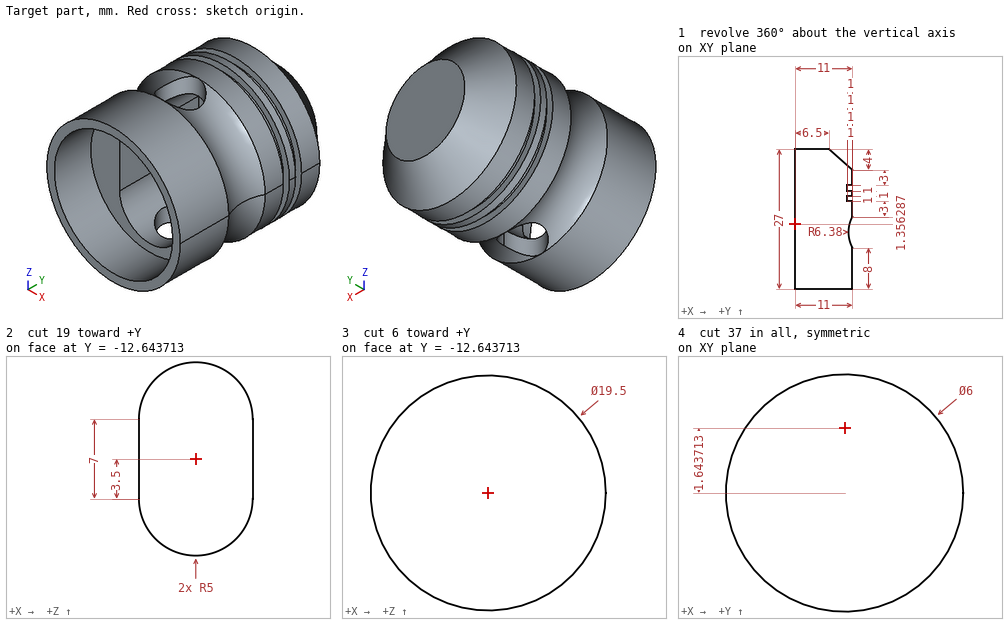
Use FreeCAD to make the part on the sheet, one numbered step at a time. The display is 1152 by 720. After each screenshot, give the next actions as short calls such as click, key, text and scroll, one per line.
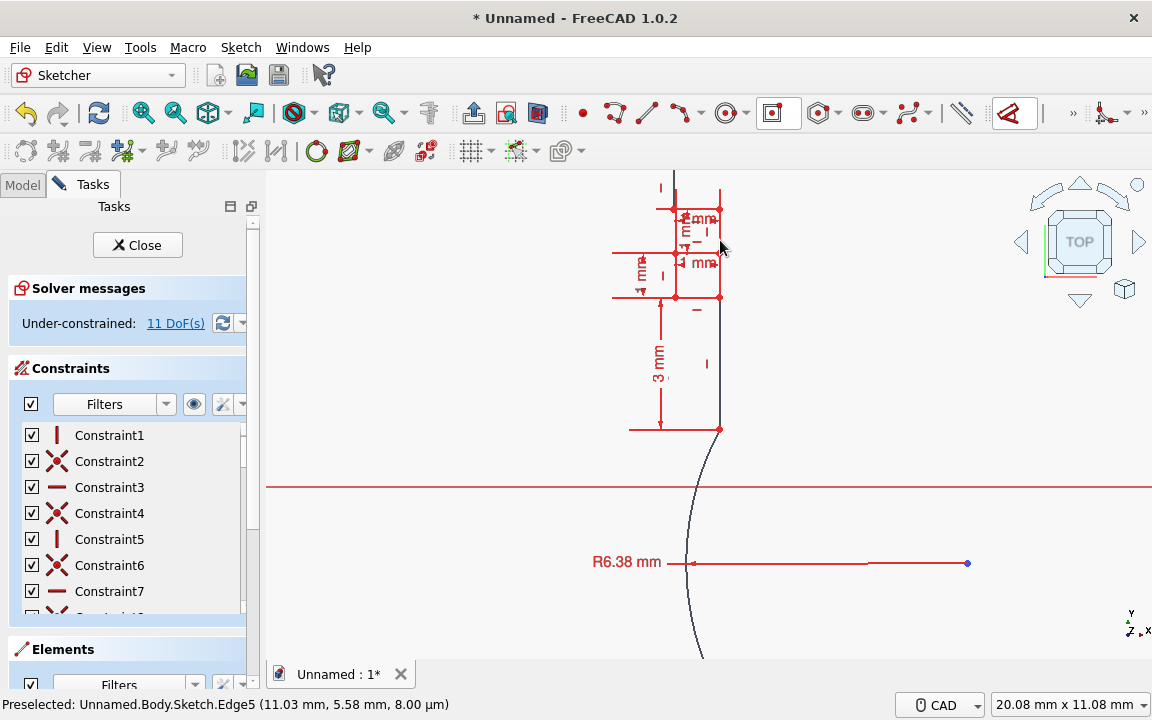
click(706, 209)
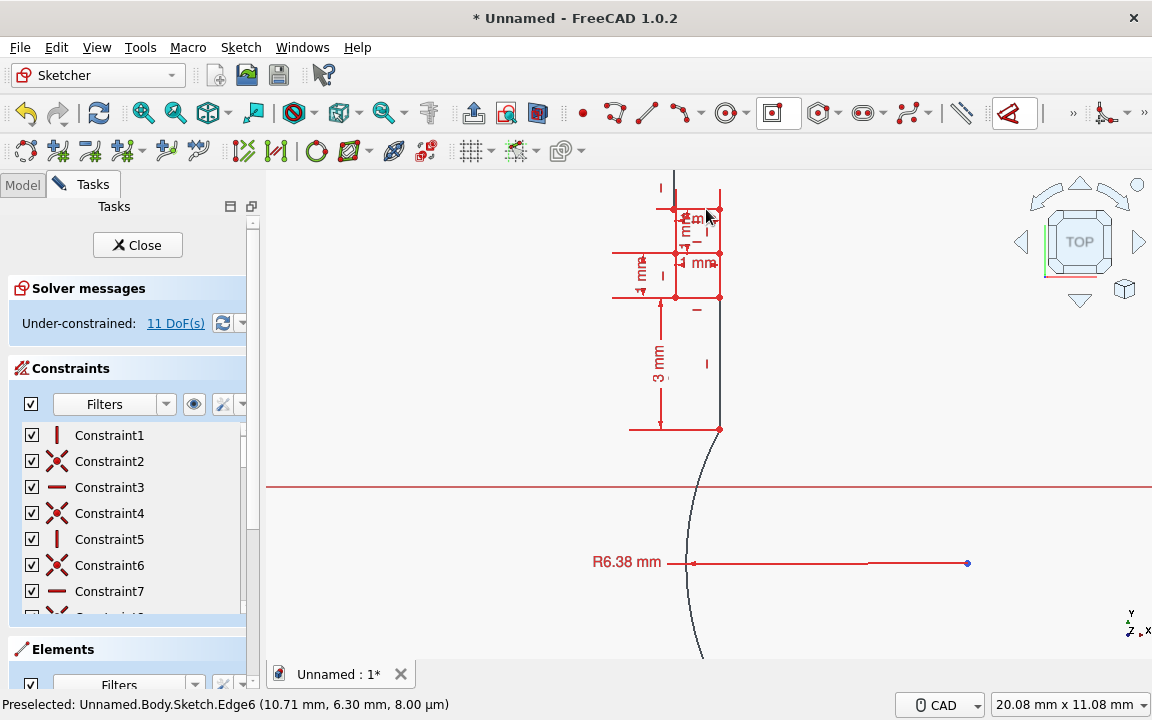
click(1032, 114)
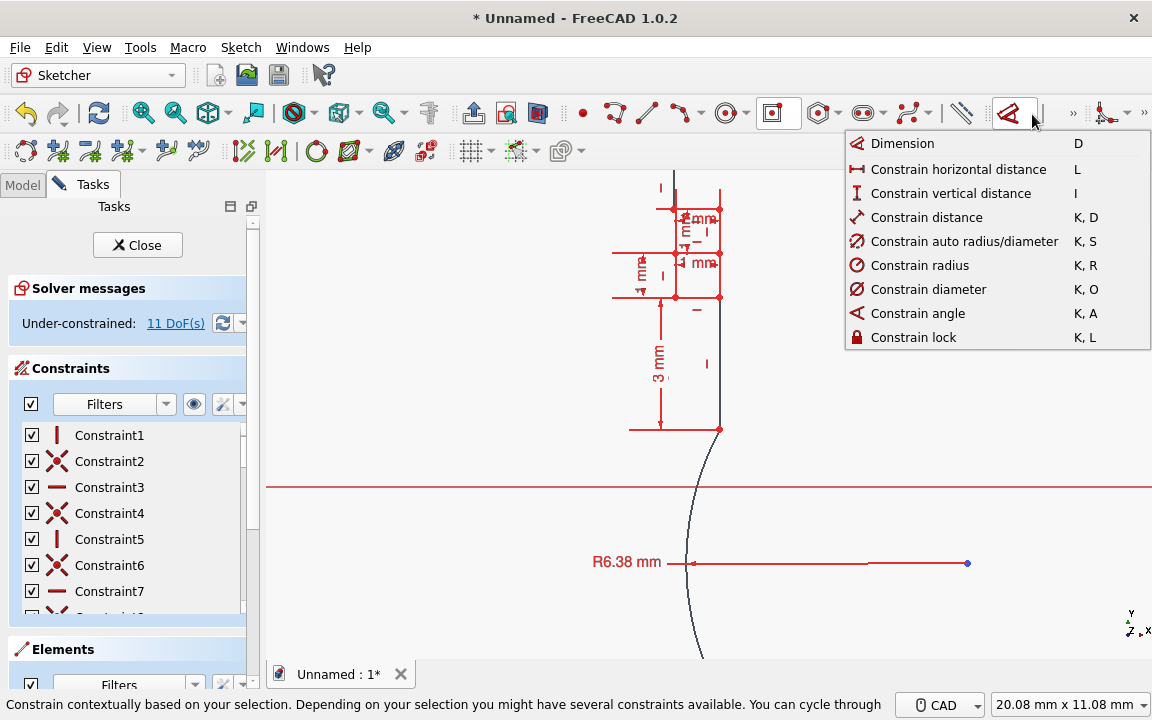
click(998, 169)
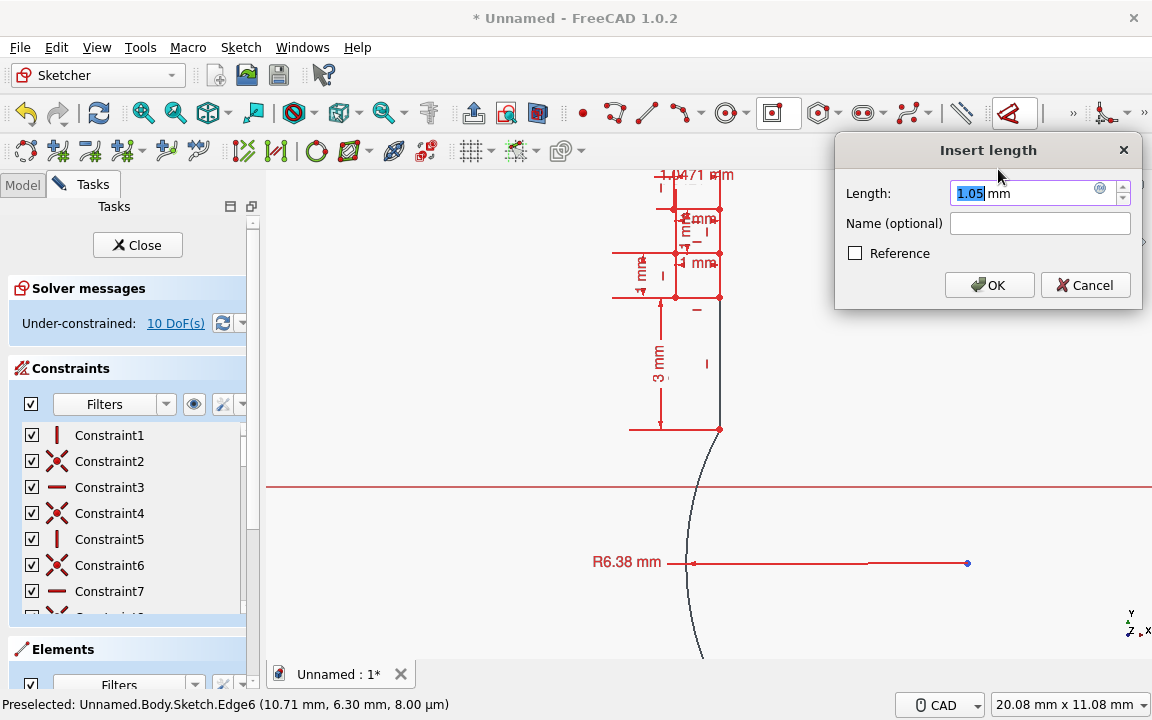
text(1)
key(Return)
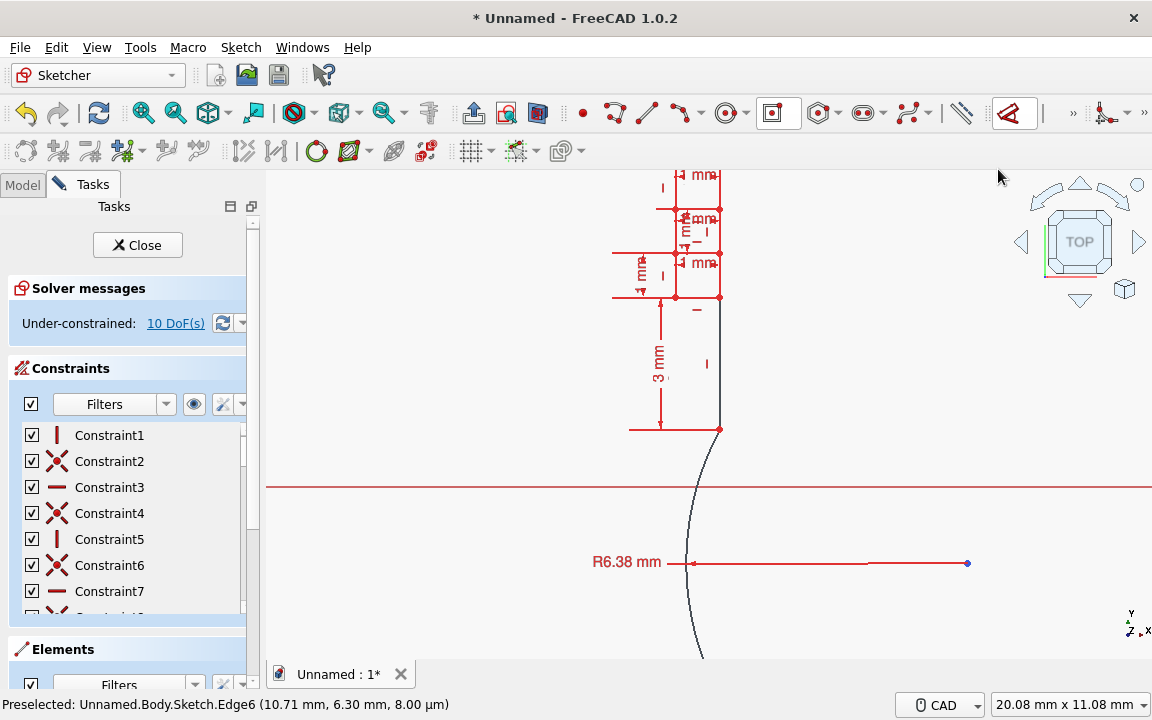
scroll(694, 403, down, 7)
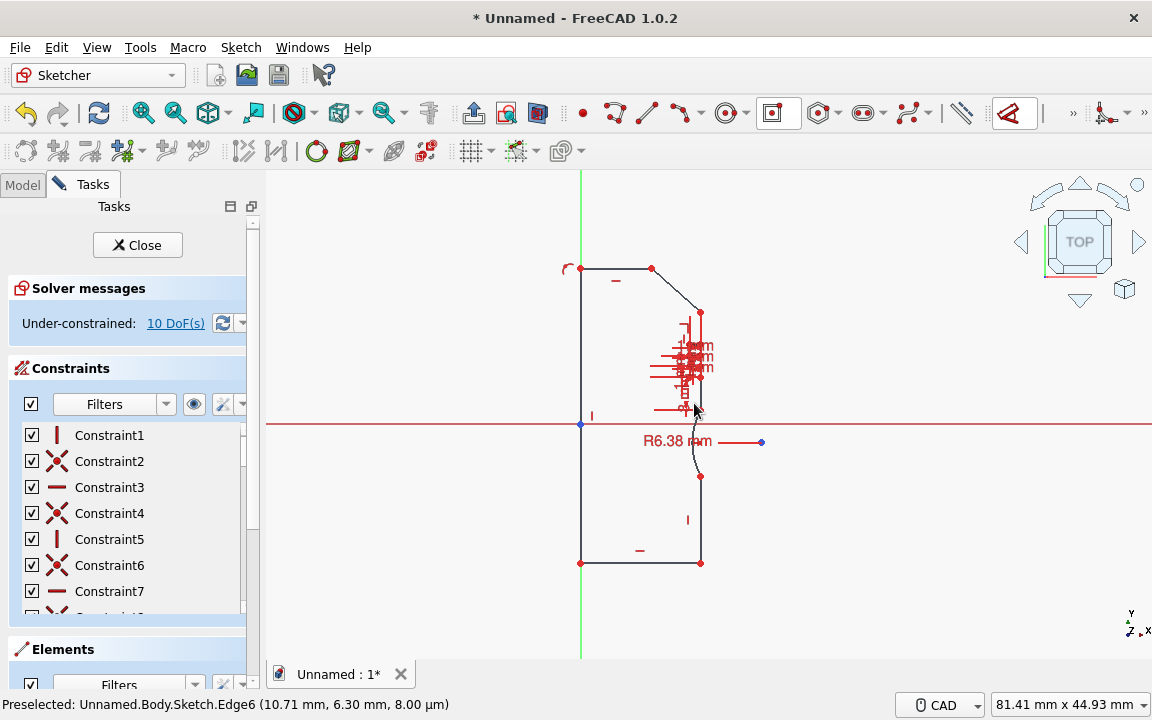
scroll(690, 352, up, 8)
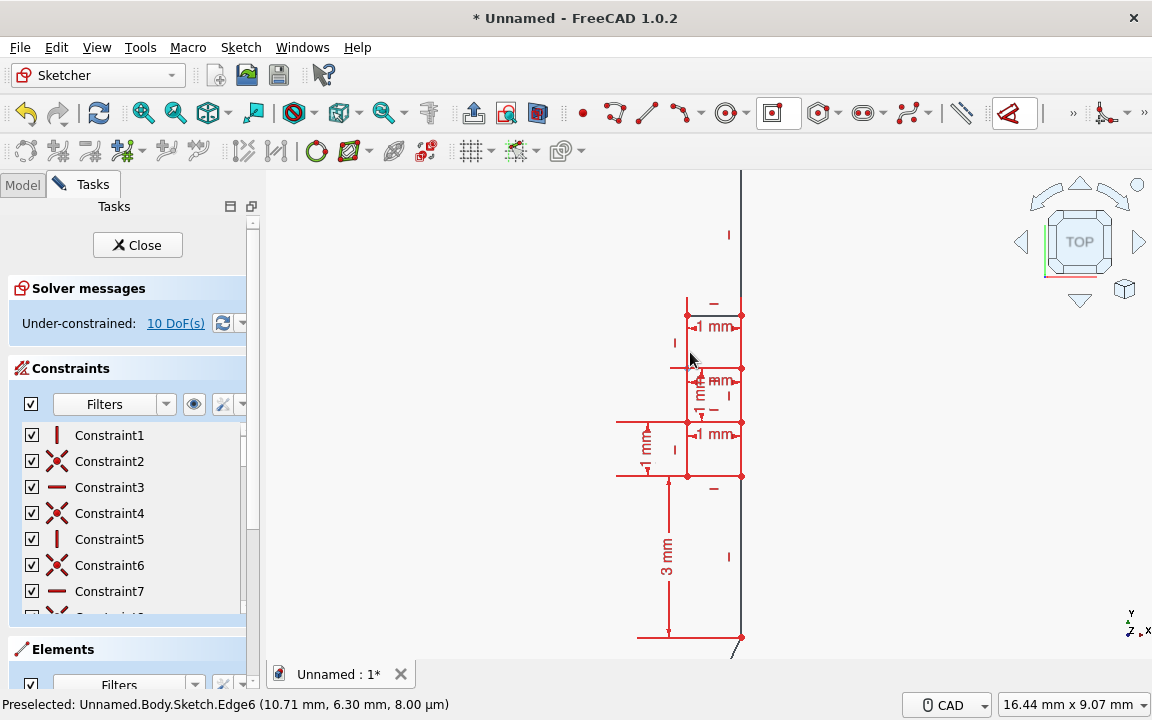
click(687, 353)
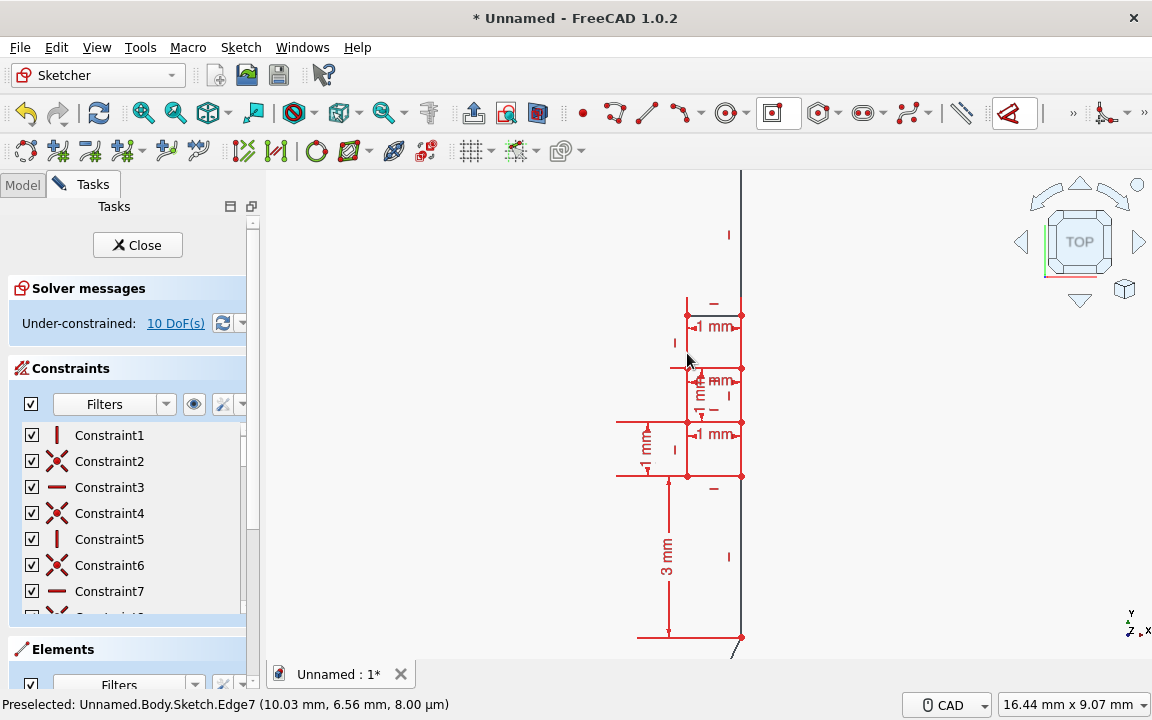
click(1032, 114)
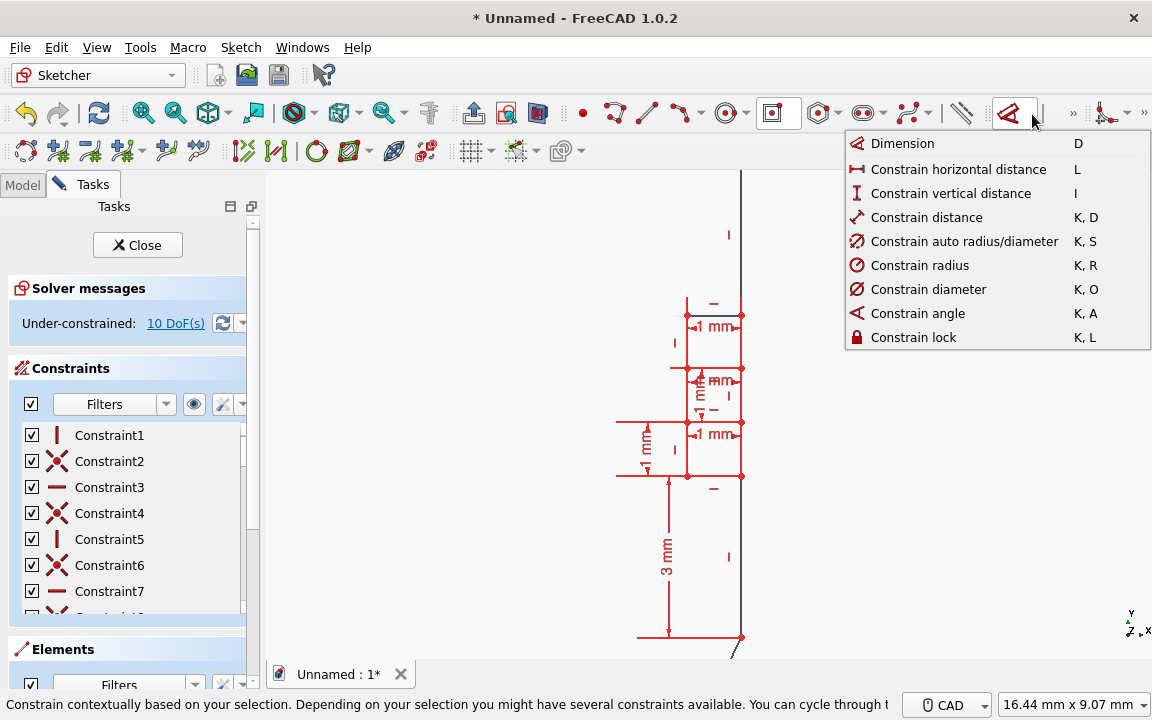
click(998, 193)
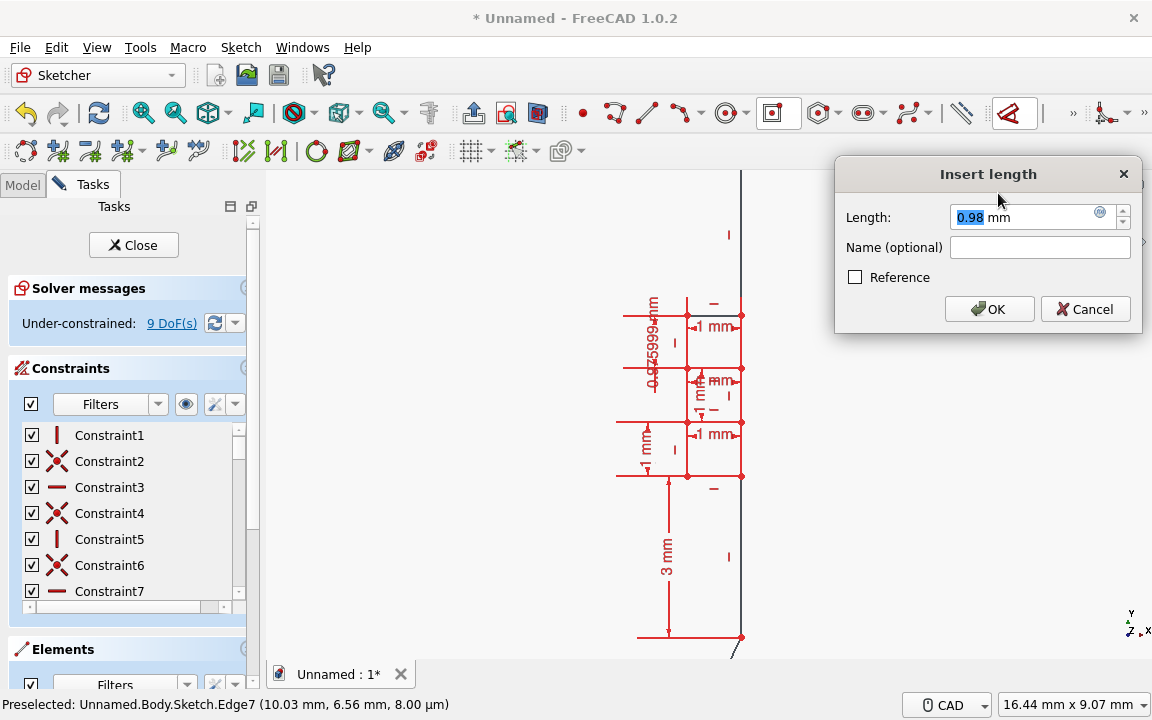
text(1)
key(Return)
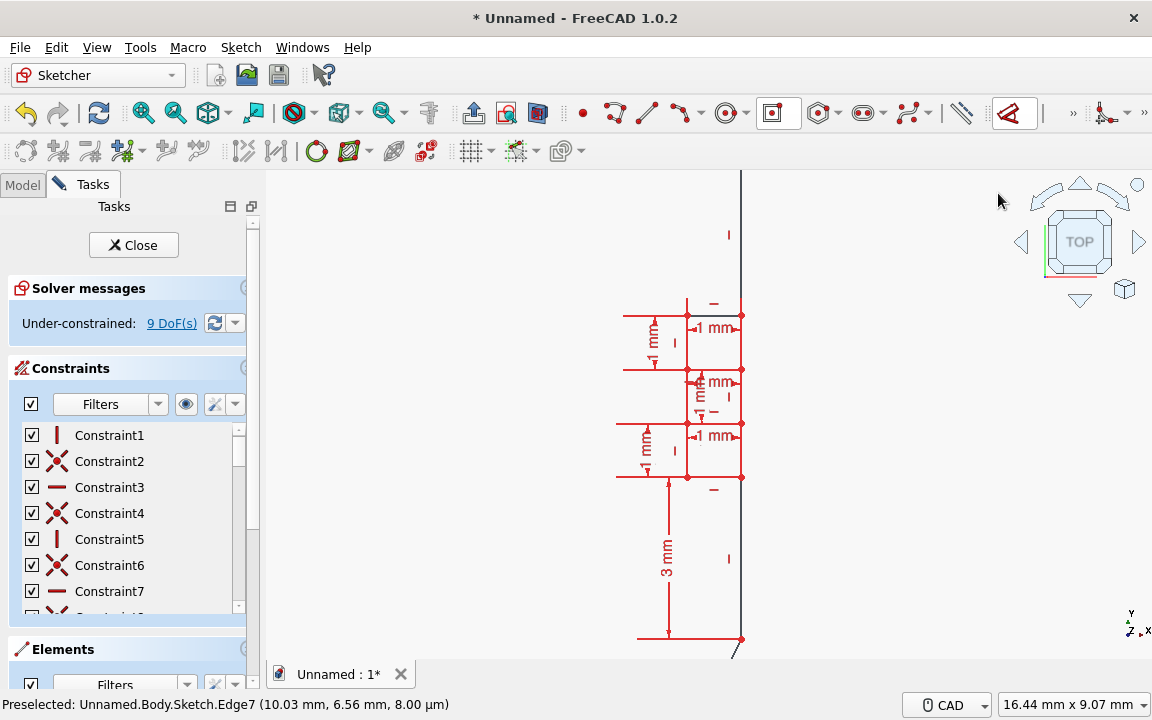
click(704, 316)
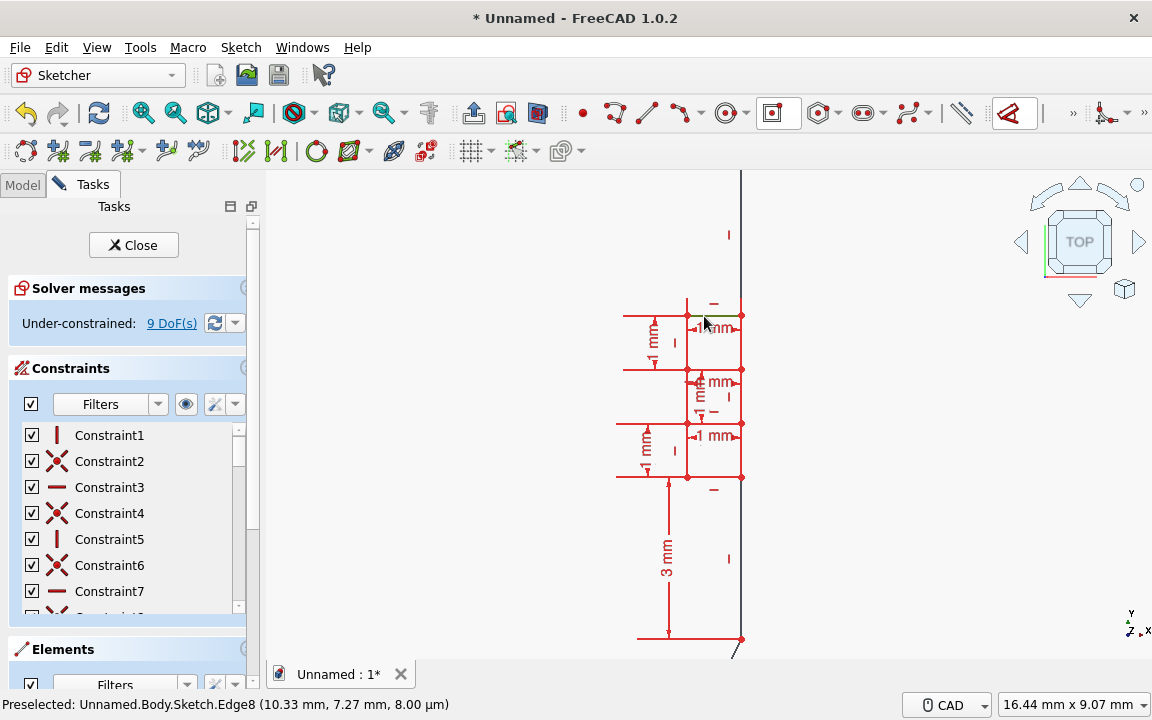
key(l)